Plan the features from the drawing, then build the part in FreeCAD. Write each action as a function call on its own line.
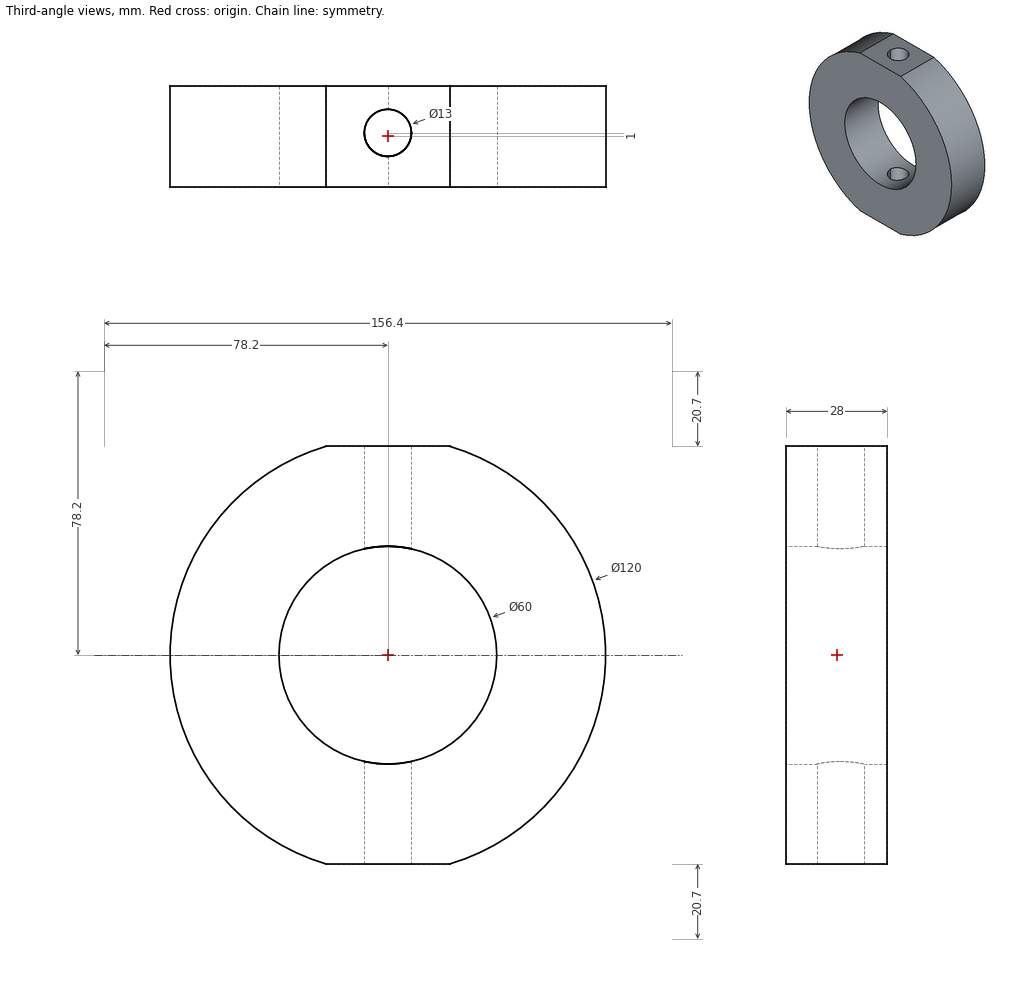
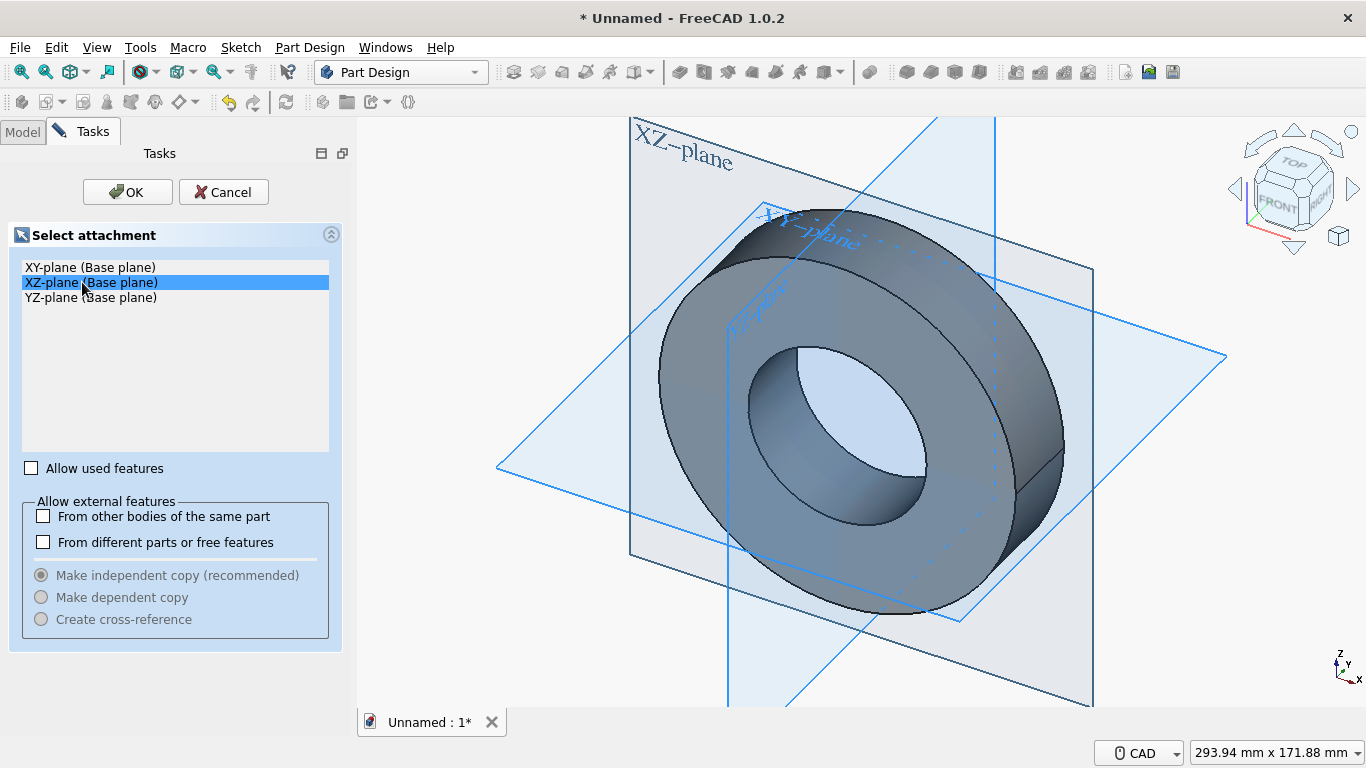
click(128, 192)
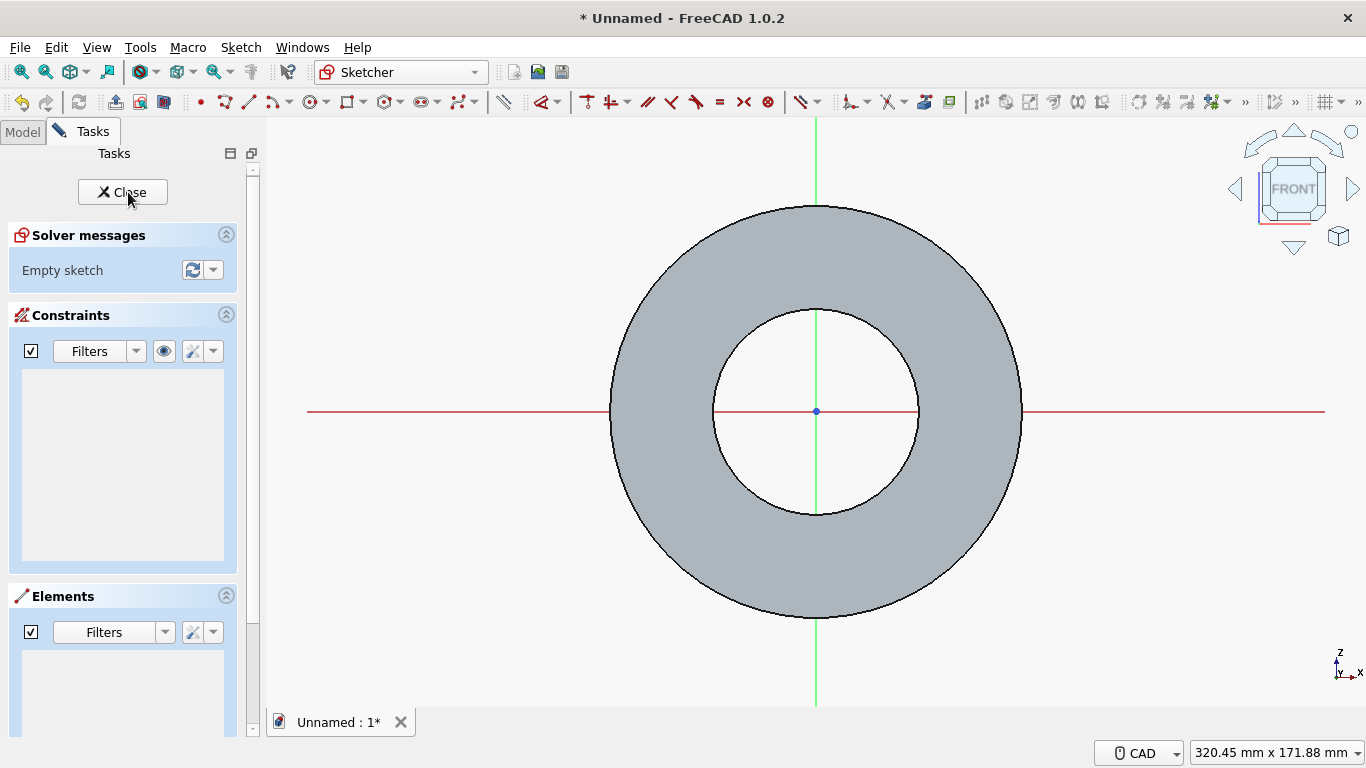
key(q)
key(s)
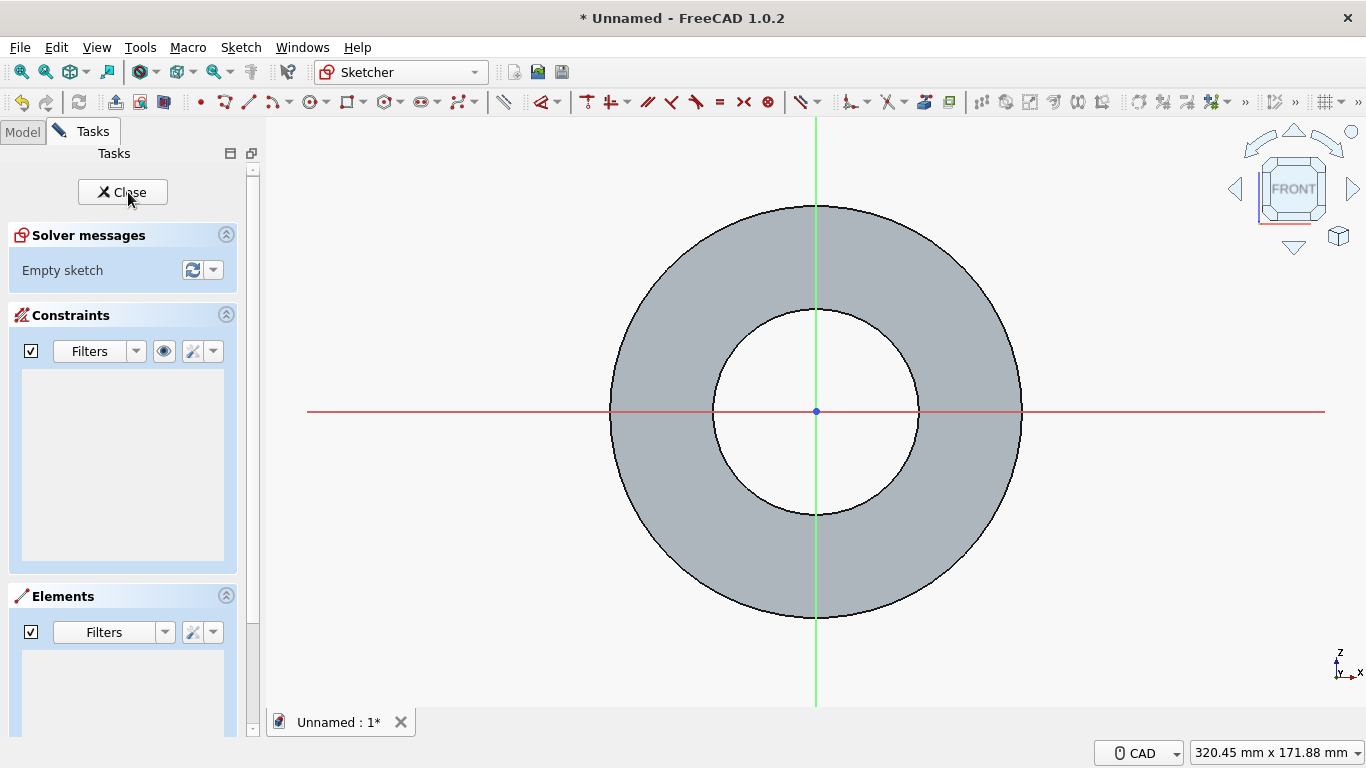
scroll(608, 412, down, 2)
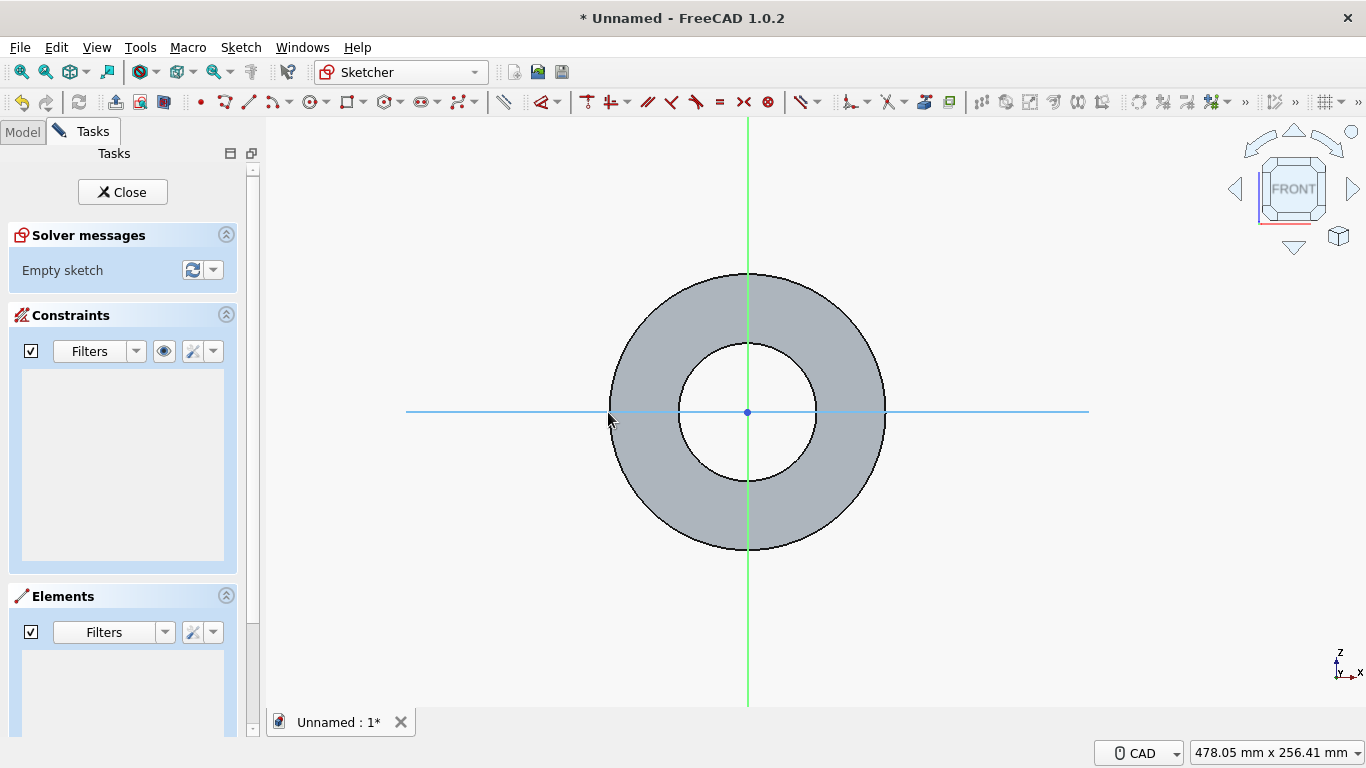
click(348, 102)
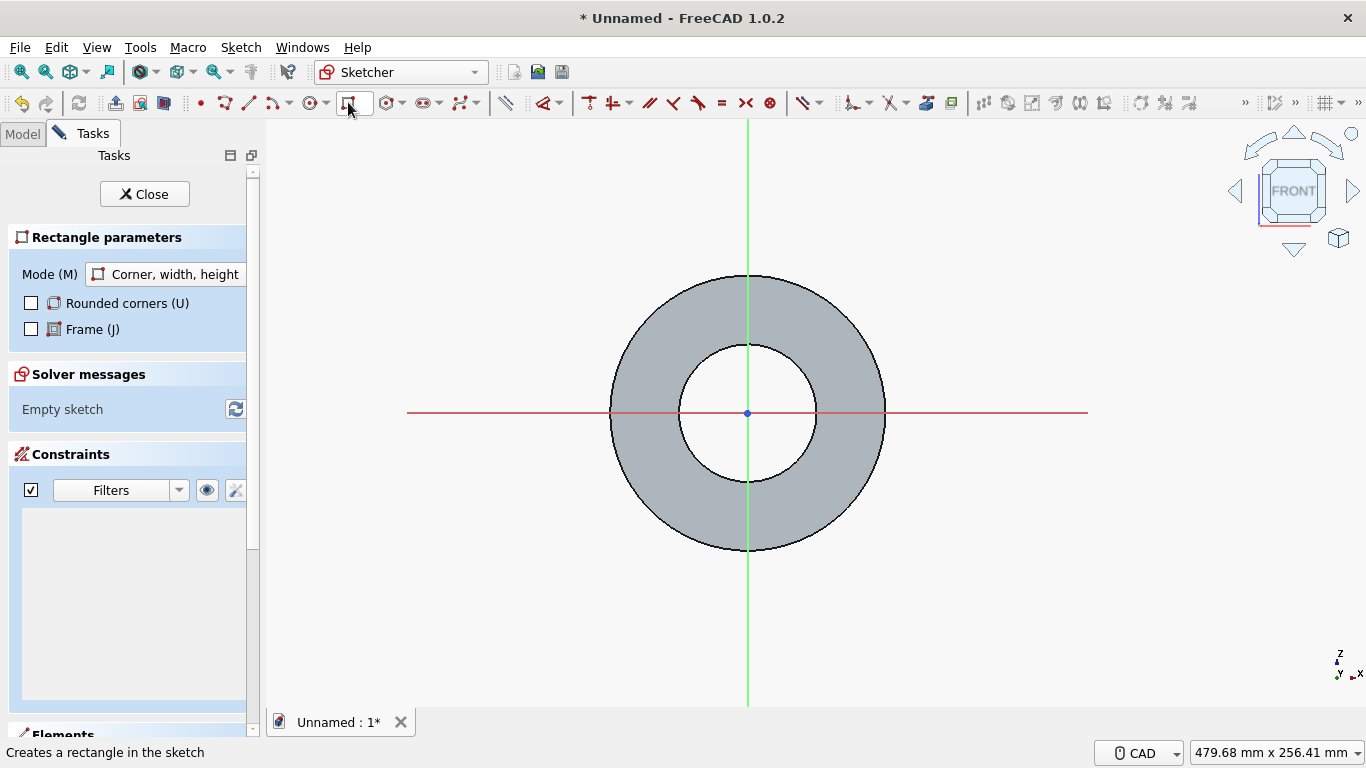
click(568, 234)
move(927, 281)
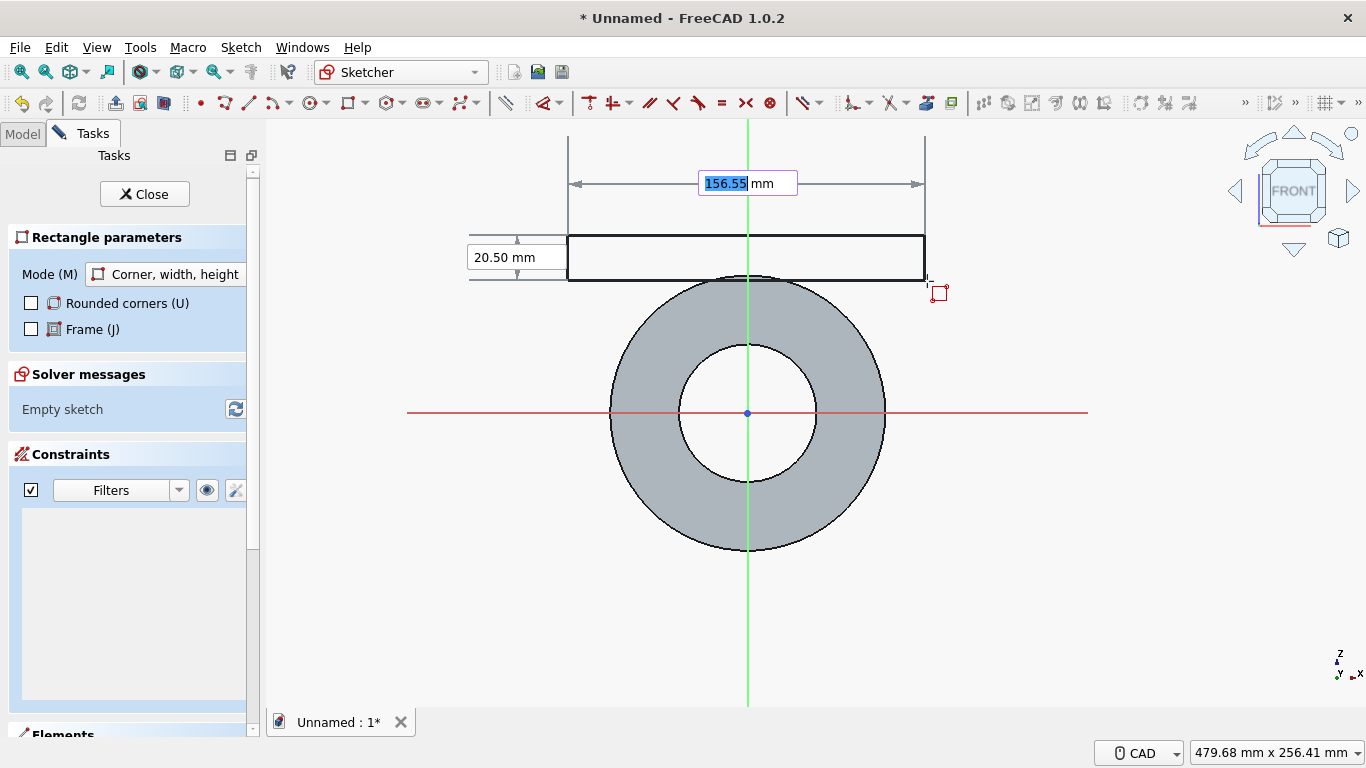
text(156.4)
key(Tab)
text(20.7)
key(Return)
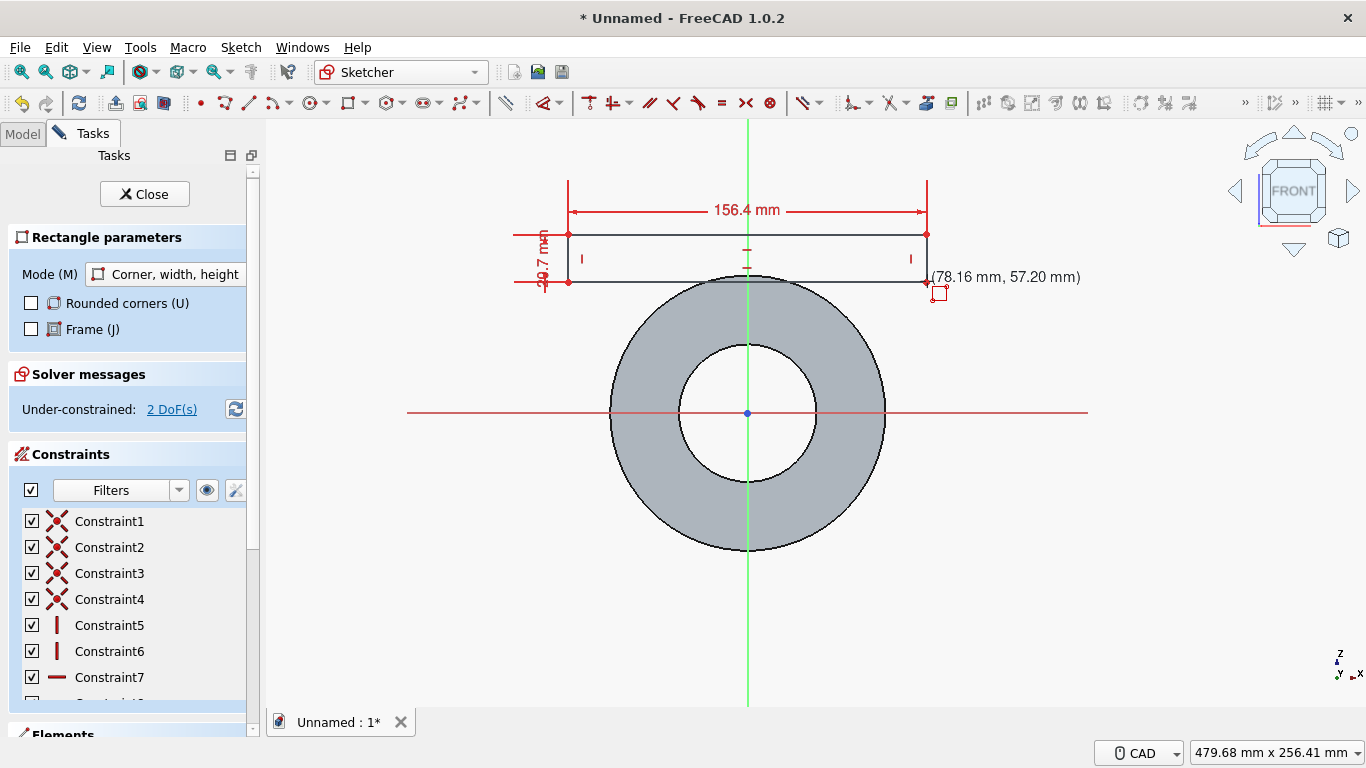
click(568, 545)
move(927, 592)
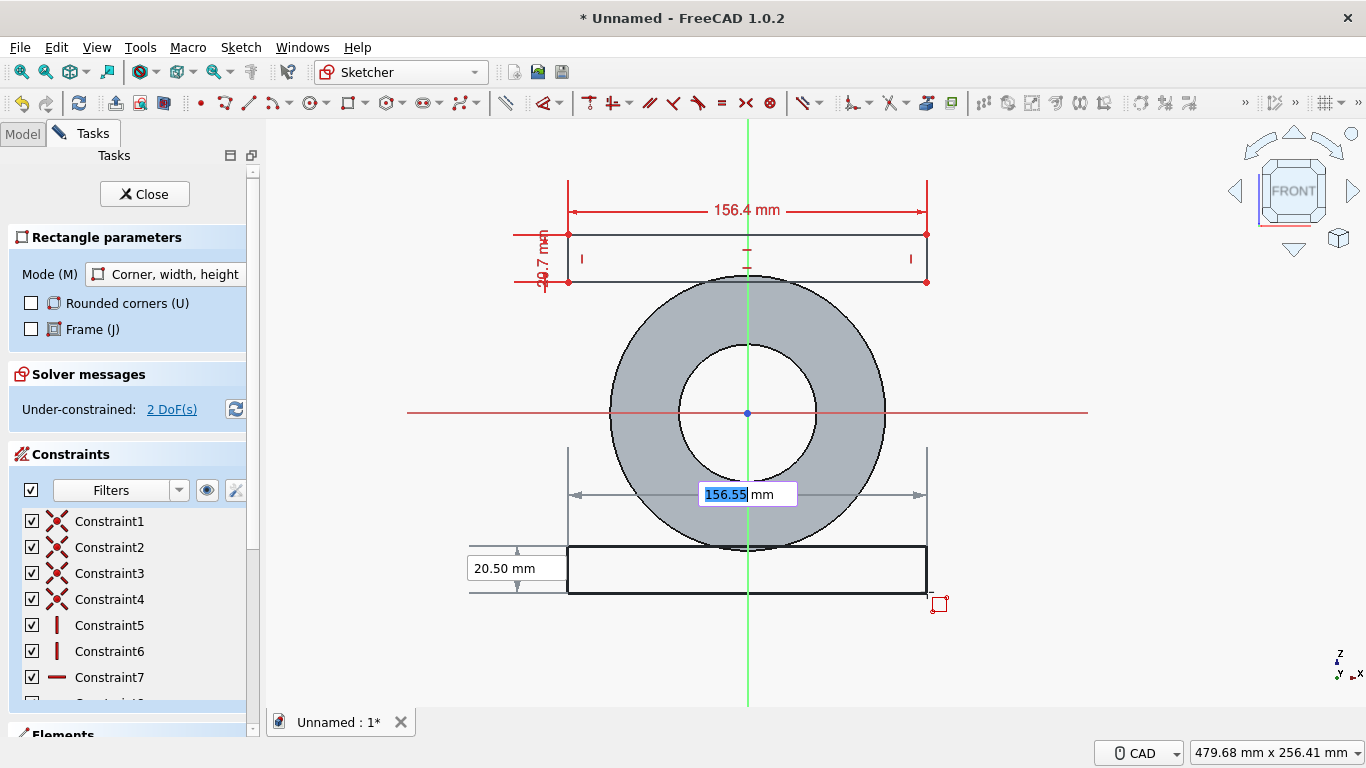
text(156.4)
key(Tab)
text(20.7)
key(Return)
key(Escape)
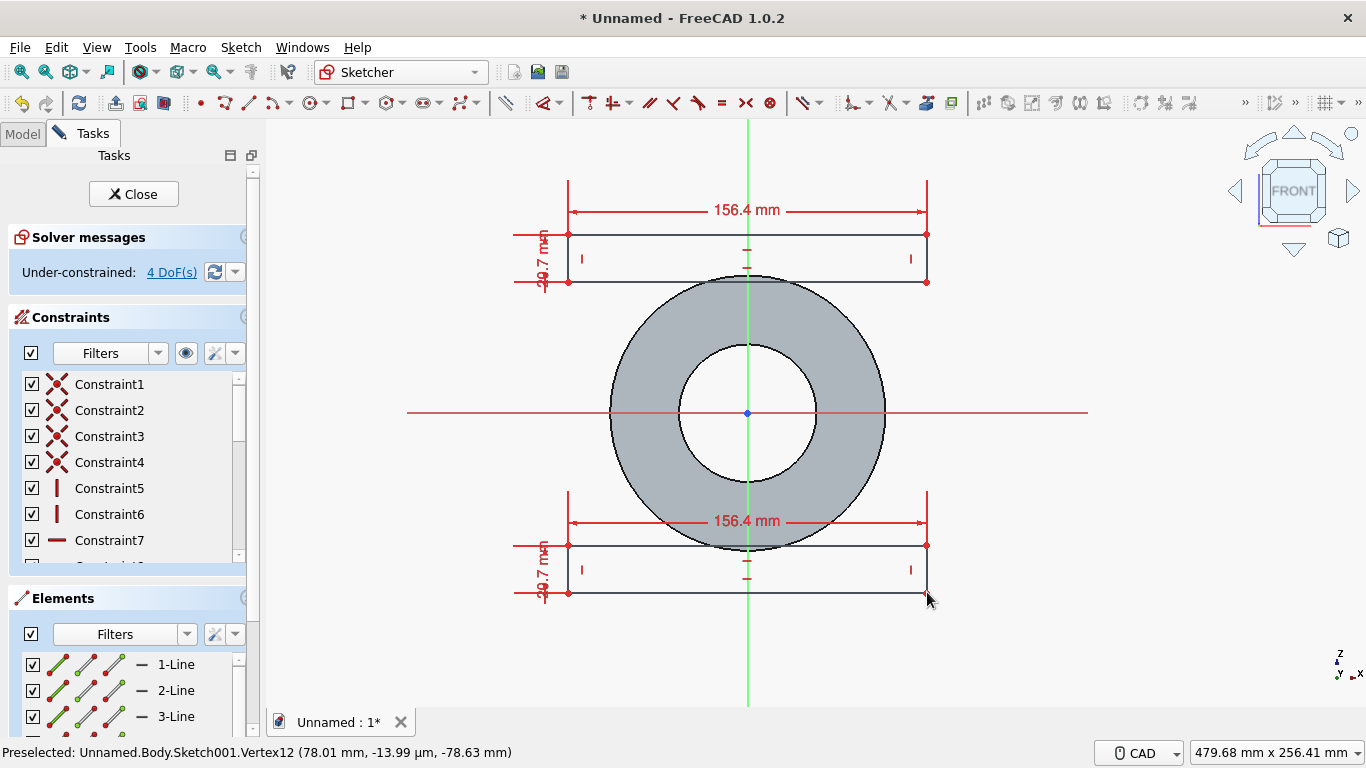
click(568, 282)